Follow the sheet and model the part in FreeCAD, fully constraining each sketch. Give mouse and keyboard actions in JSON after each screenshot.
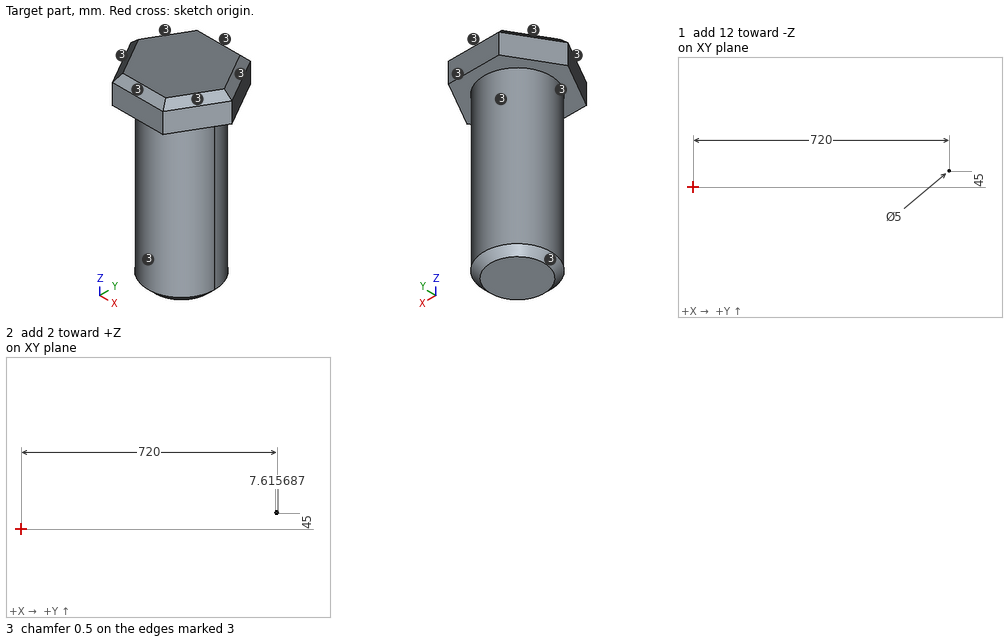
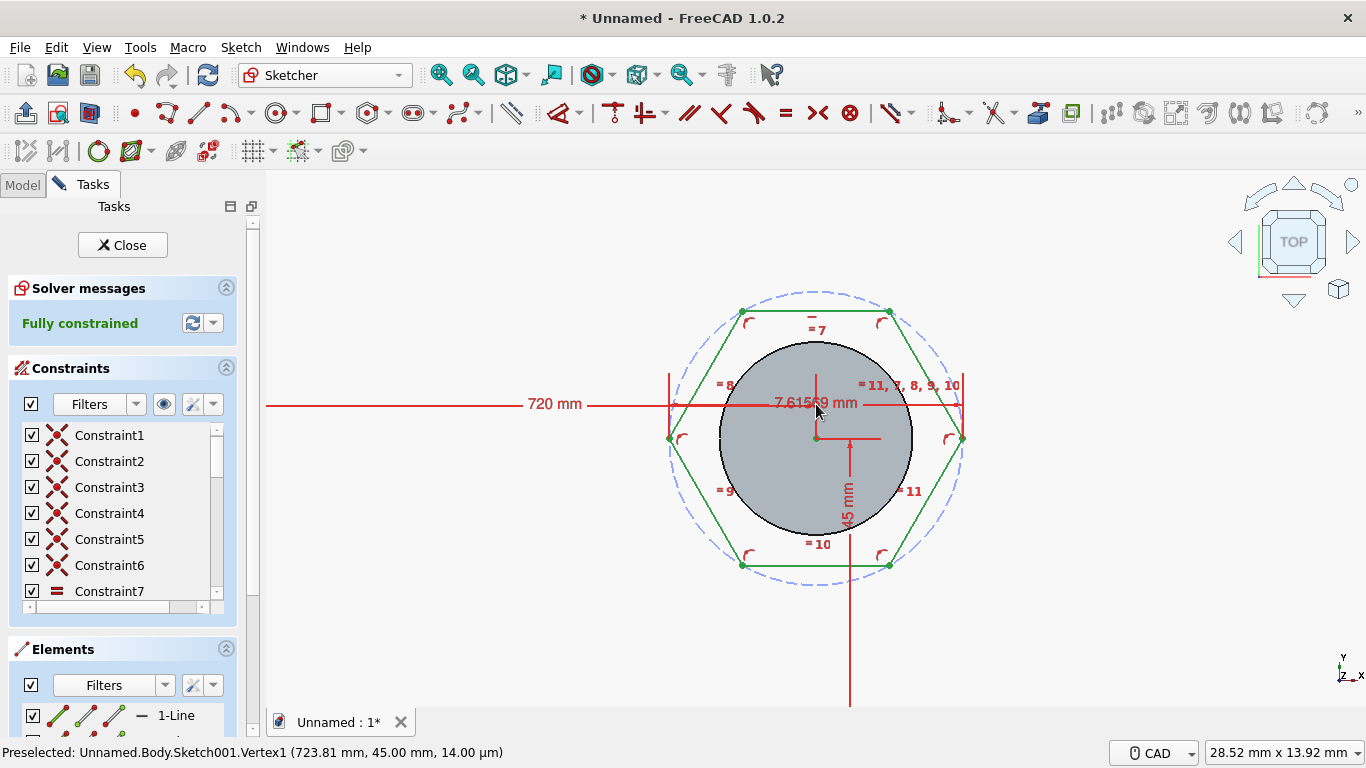
{"action": "left_click", "coordinate": [123, 245]}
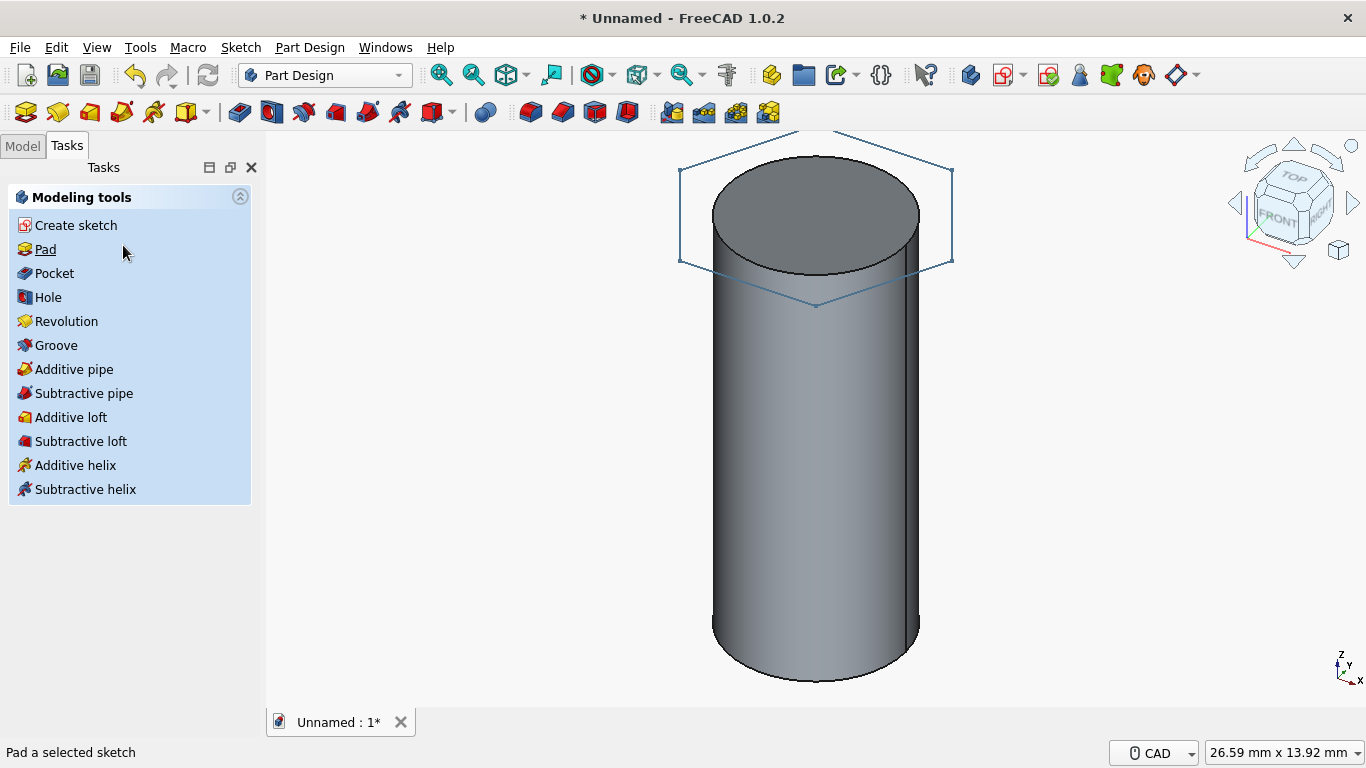
{"action": "left_click", "coordinate": [26, 112]}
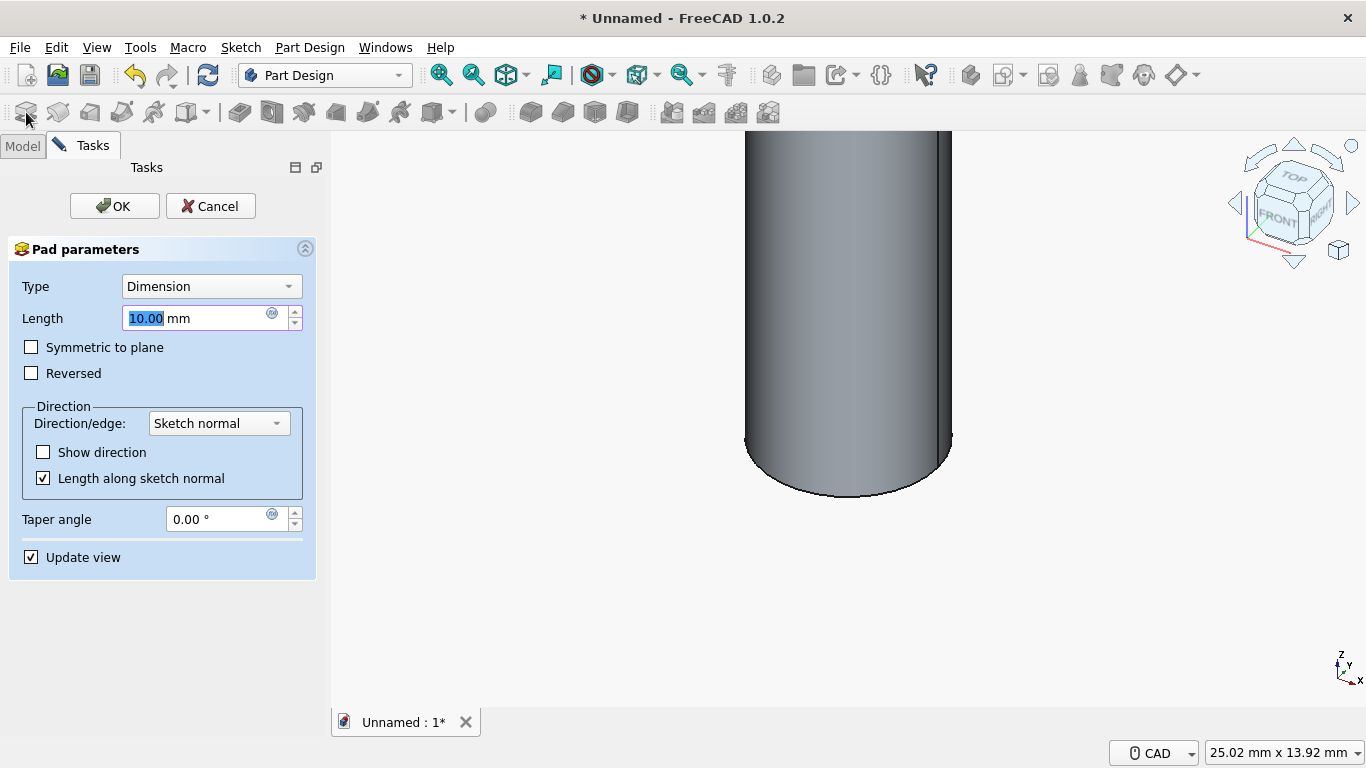
{"action": "type", "text": "2"}
{"action": "key", "text": "Tab"}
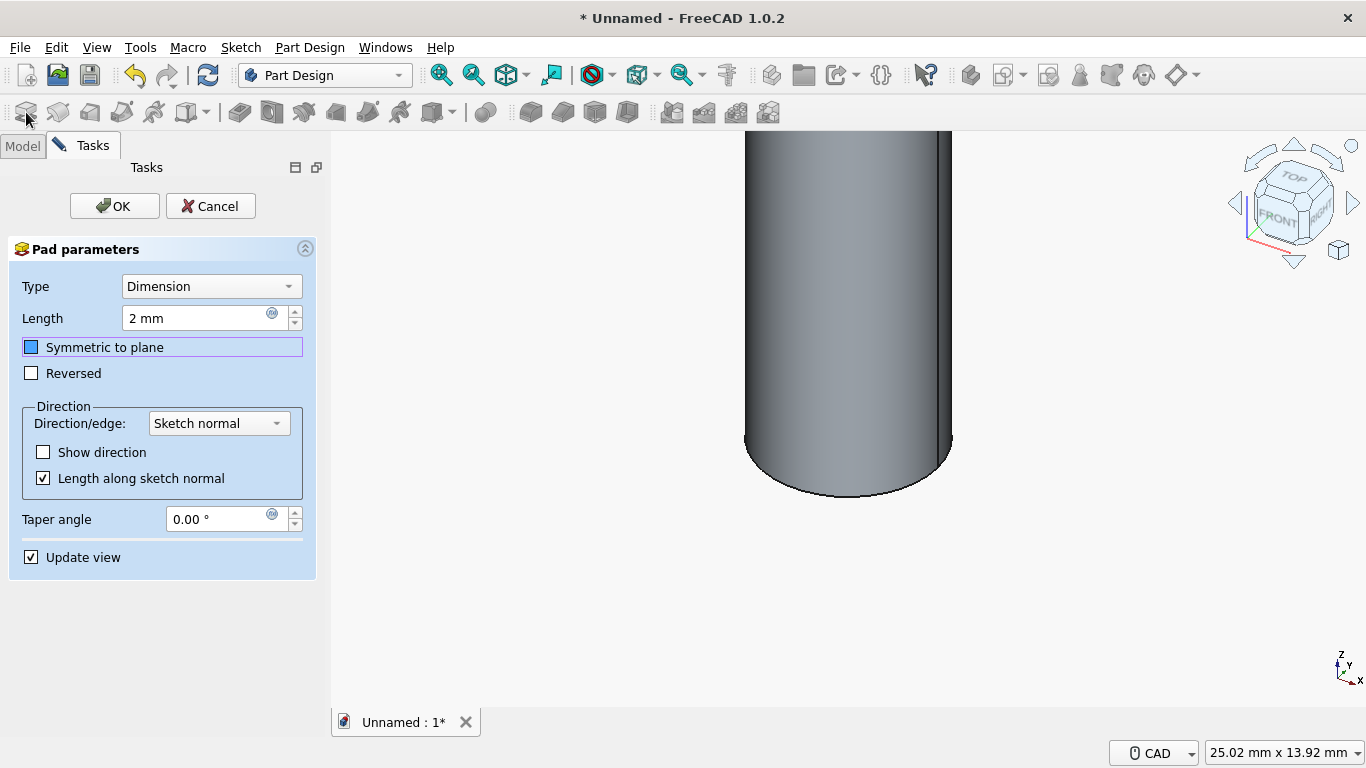
{"action": "left_click", "coordinate": [115, 206]}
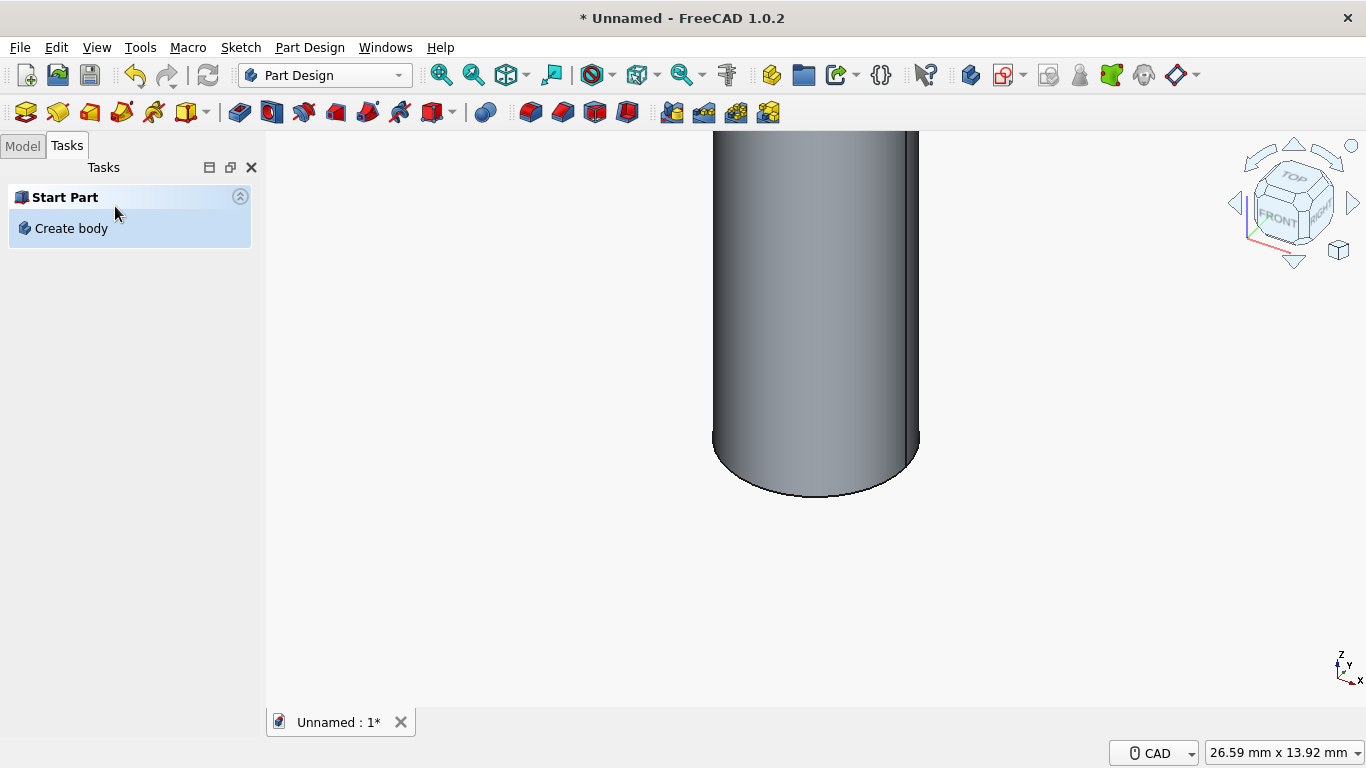
{"action": "left_click", "coordinate": [442, 76]}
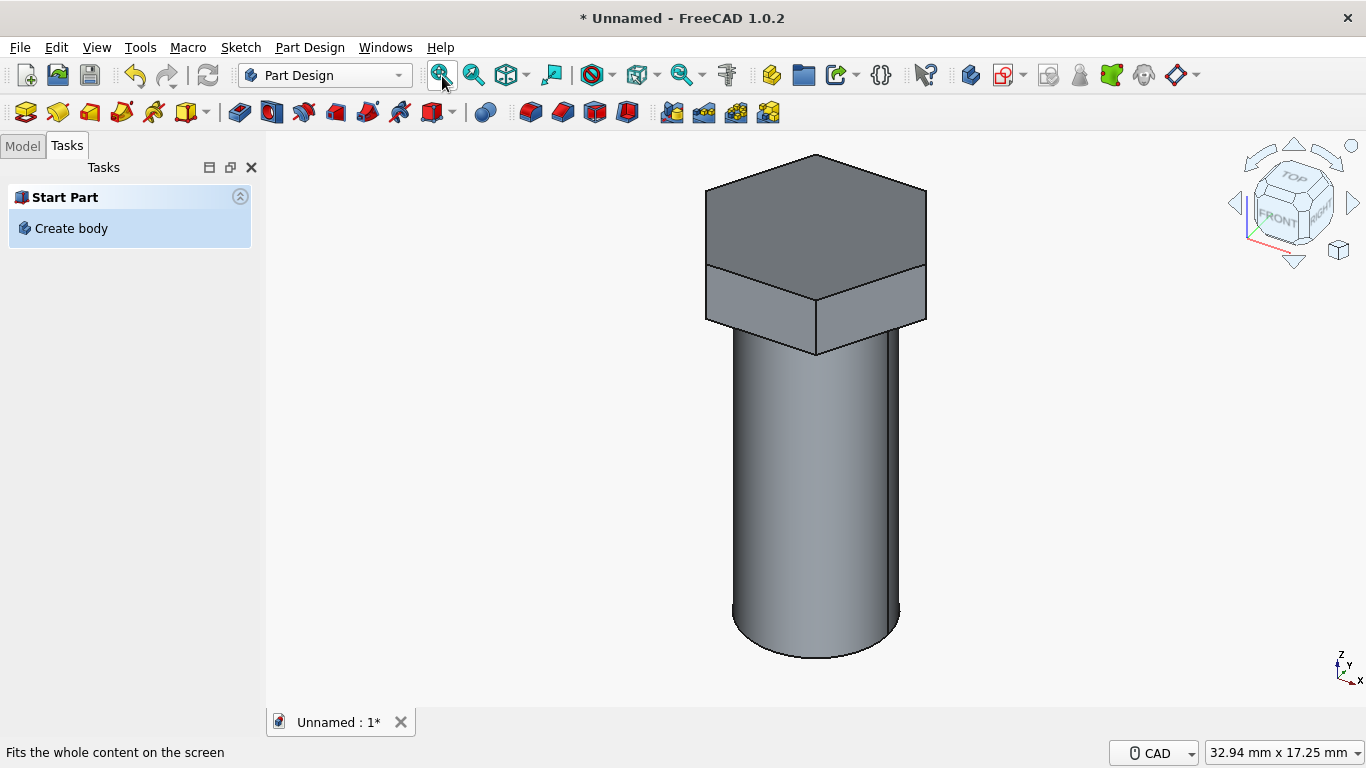
{"action": "left_click", "coordinate": [816, 227]}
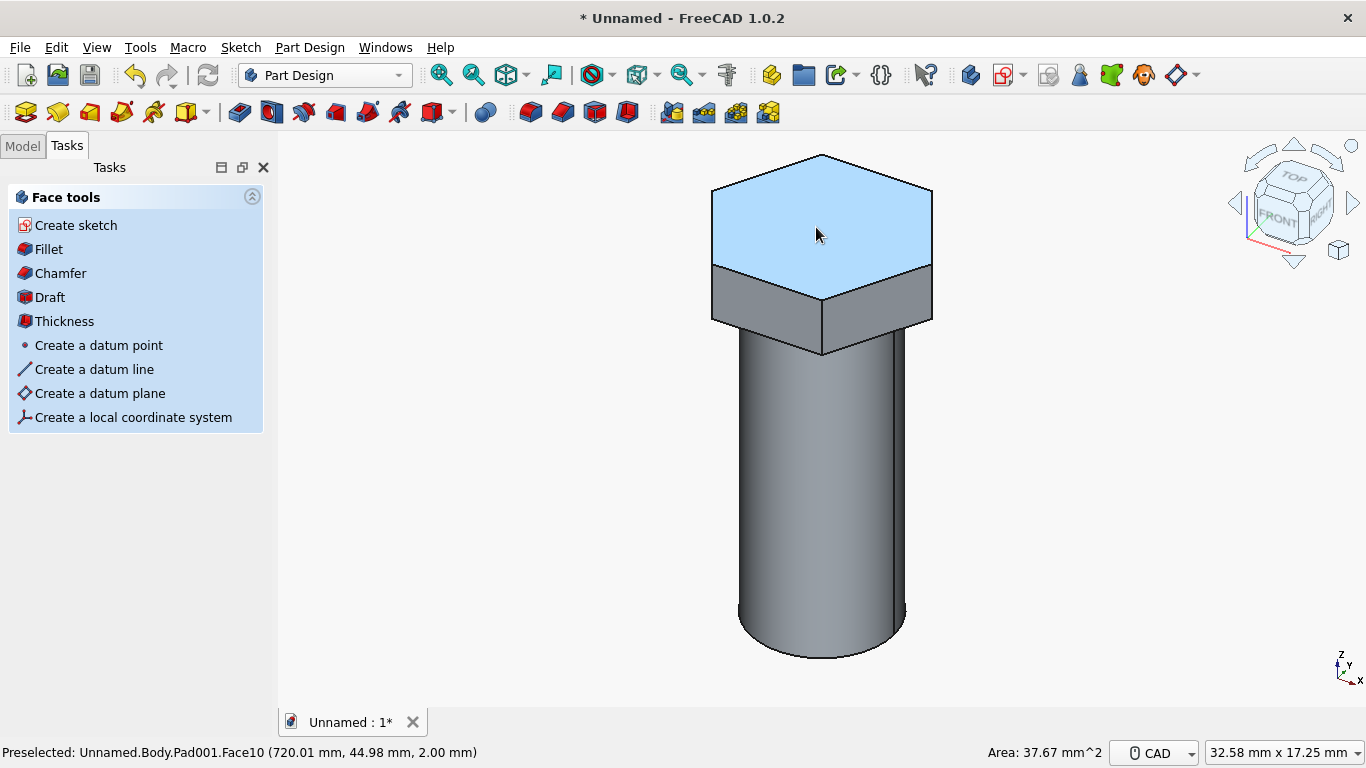
{"action": "key", "text": "0"}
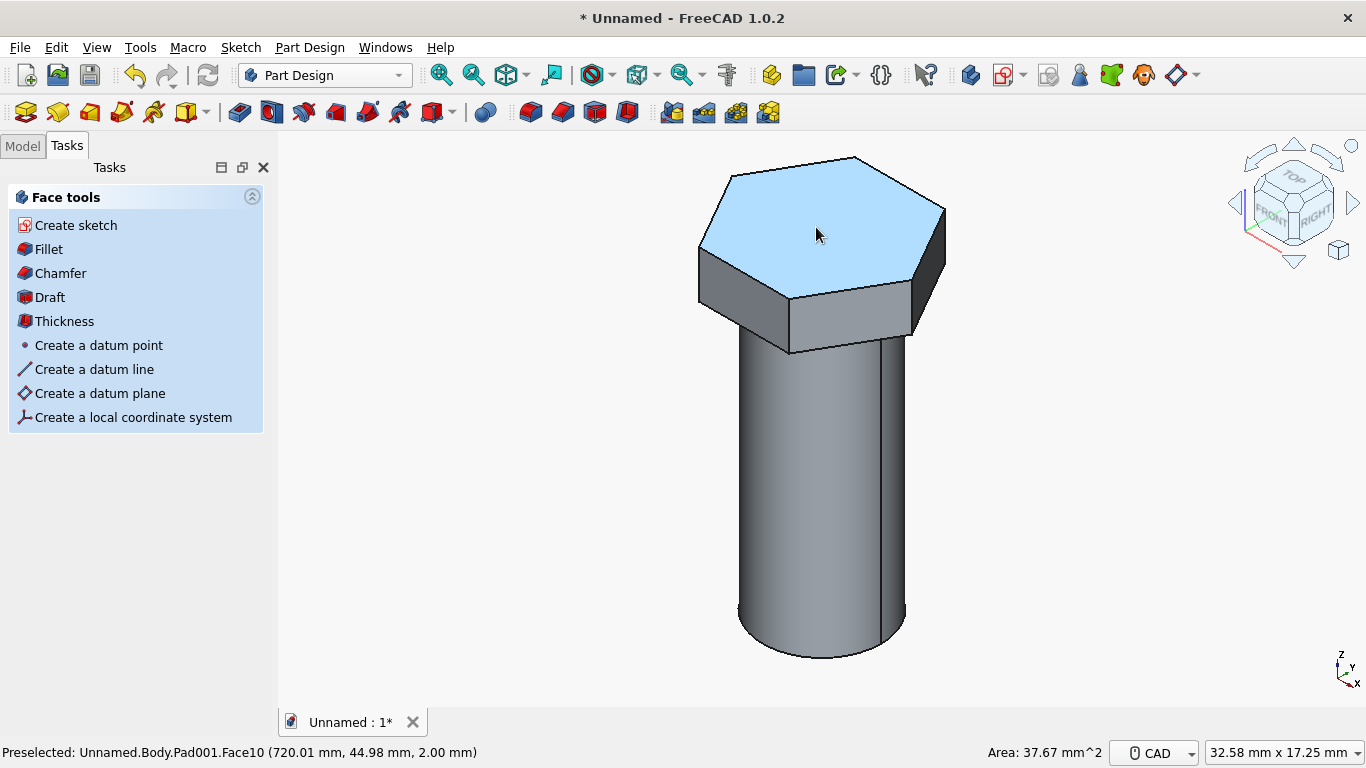
{"action": "left_click", "coordinate": [442, 76]}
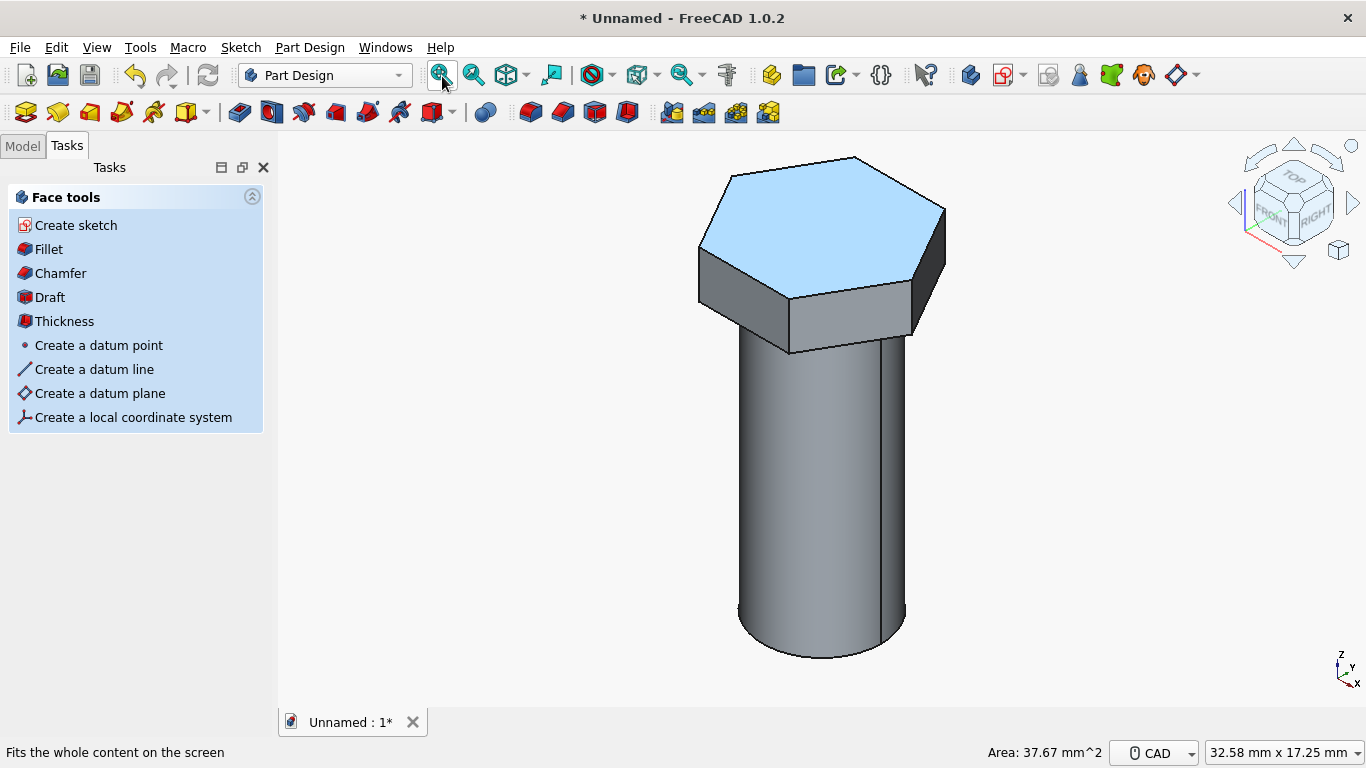
{"action": "key", "text": "2"}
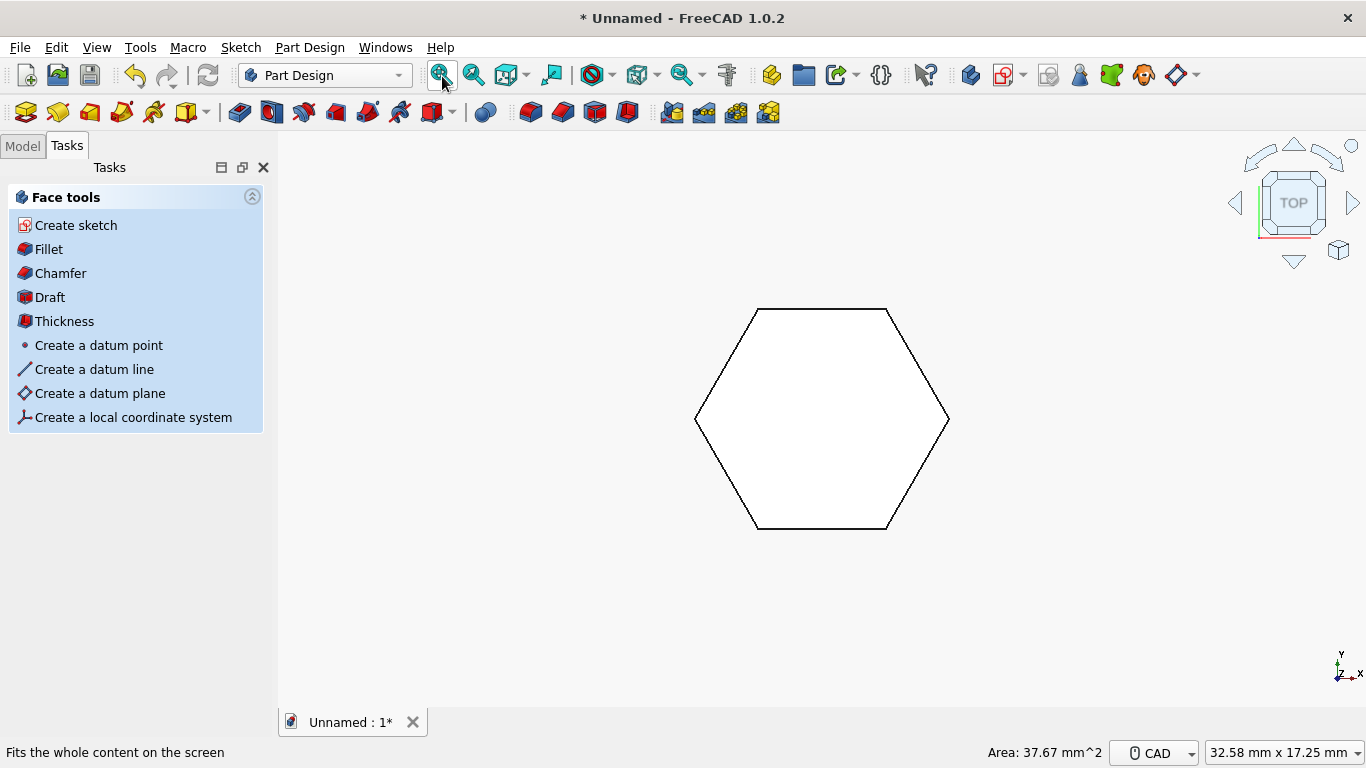
{"action": "left_click", "coordinate": [442, 76]}